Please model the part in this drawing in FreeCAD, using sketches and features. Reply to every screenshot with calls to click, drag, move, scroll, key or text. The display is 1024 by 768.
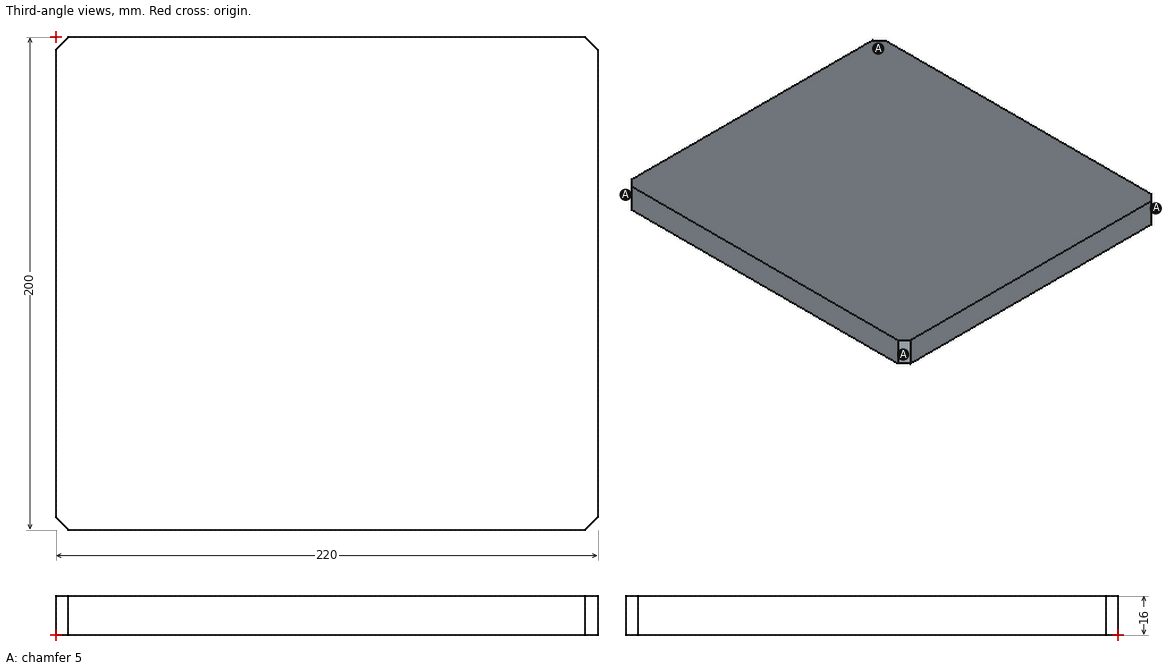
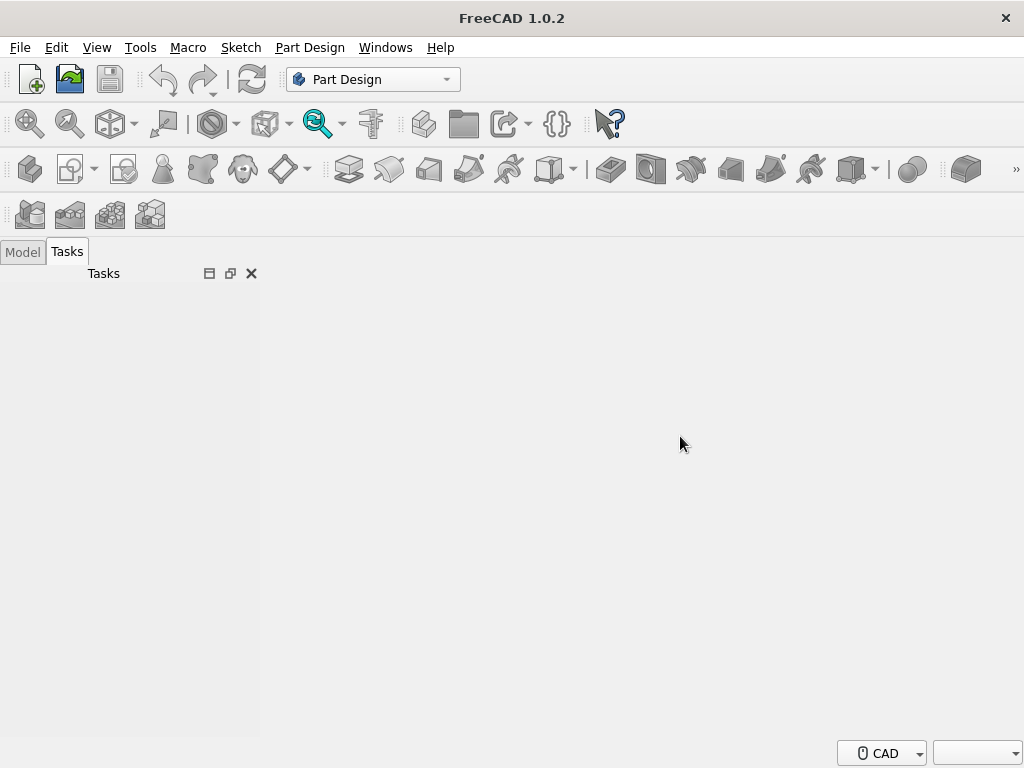
click(30, 80)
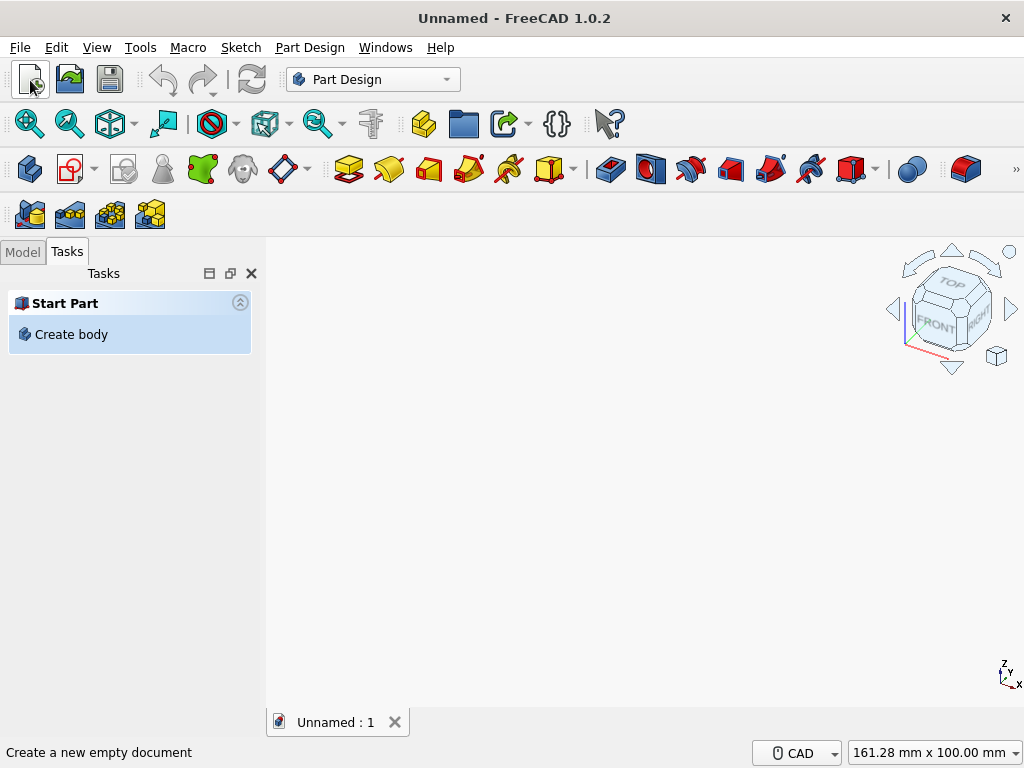
click(70, 170)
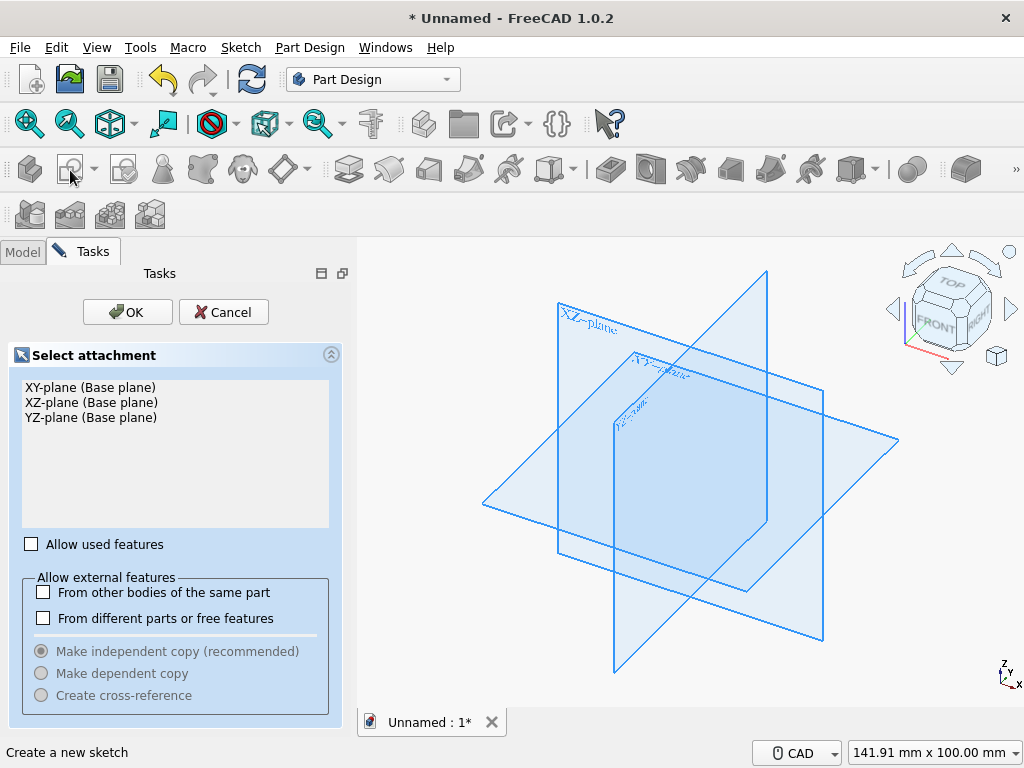
click(82, 388)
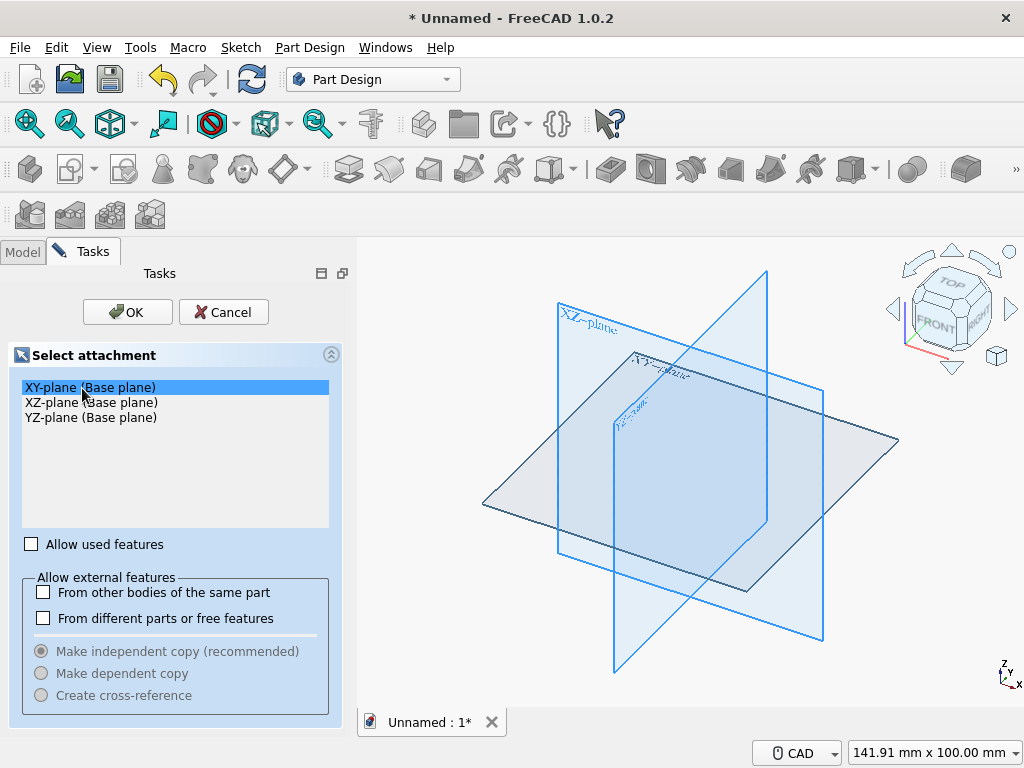
click(128, 312)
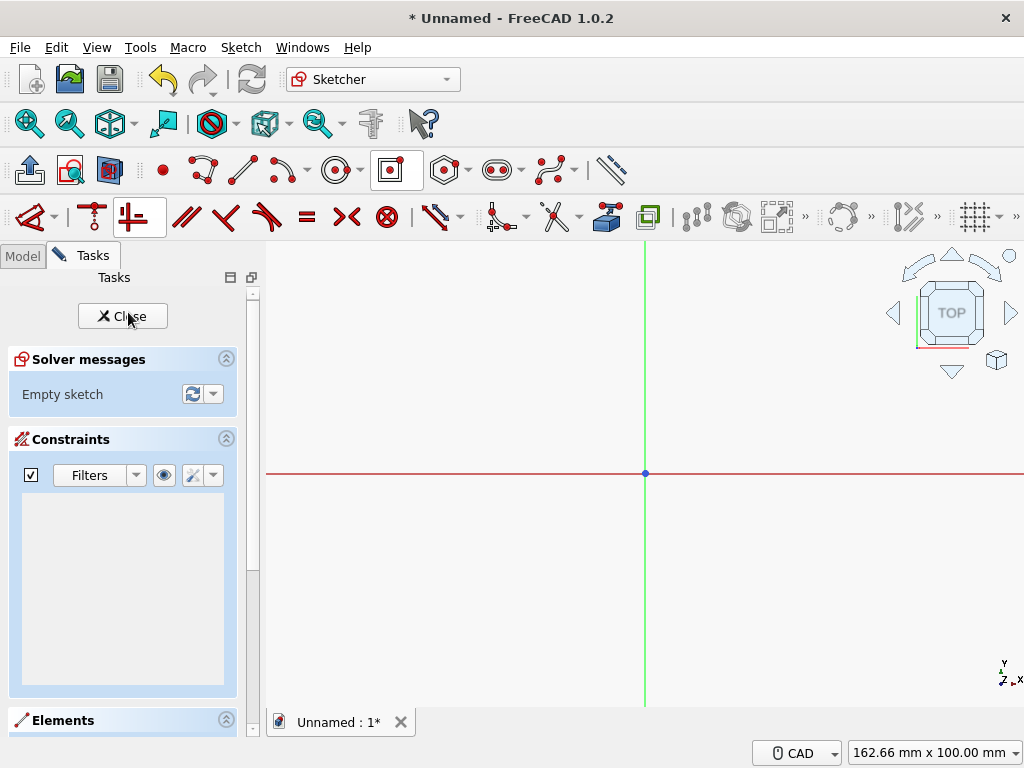
scroll(326, 273, down, 6)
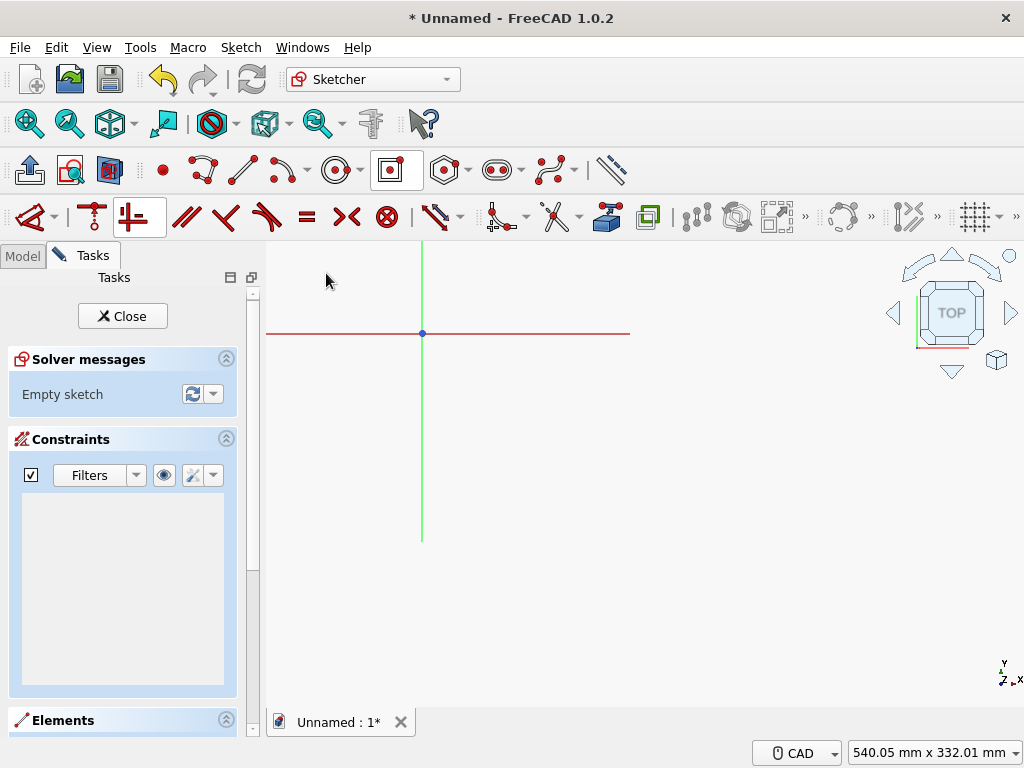
key(g)
key(r)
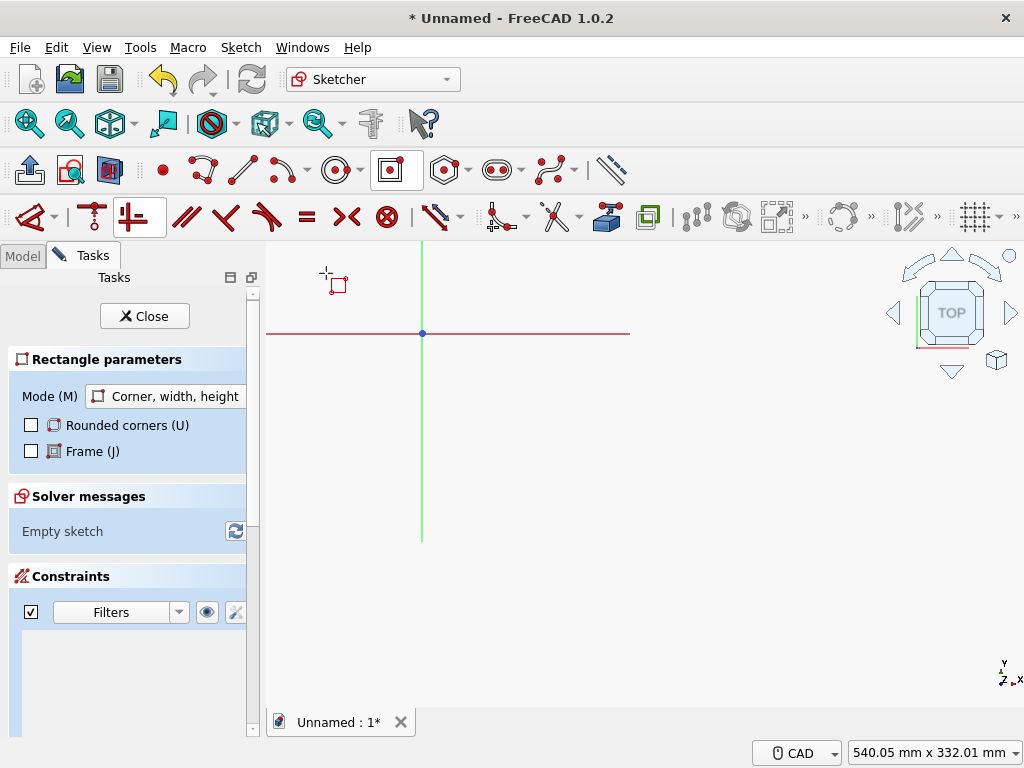
click(422, 334)
click(731, 614)
key(Escape)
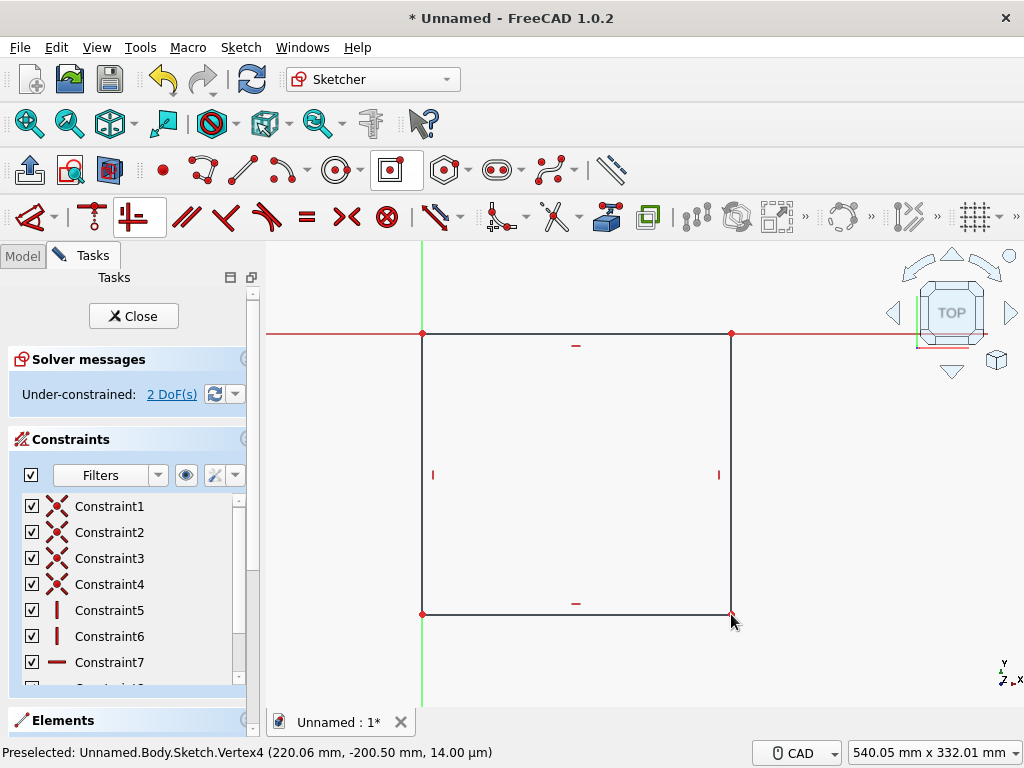
click(30, 218)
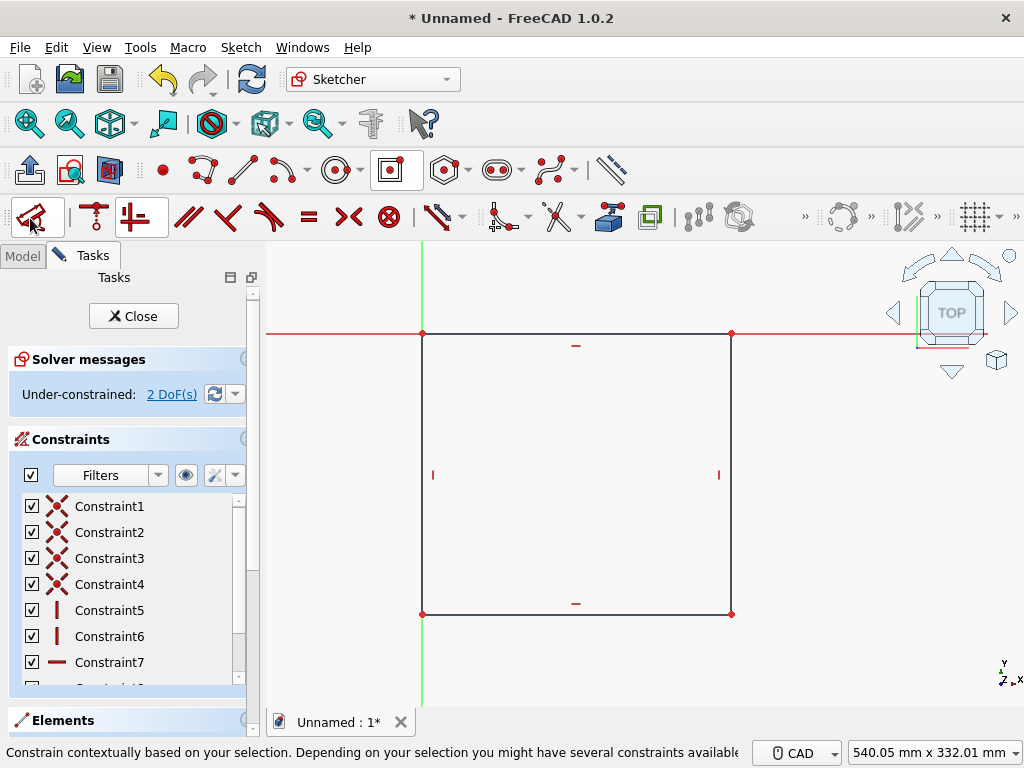
click(422, 418)
click(388, 474)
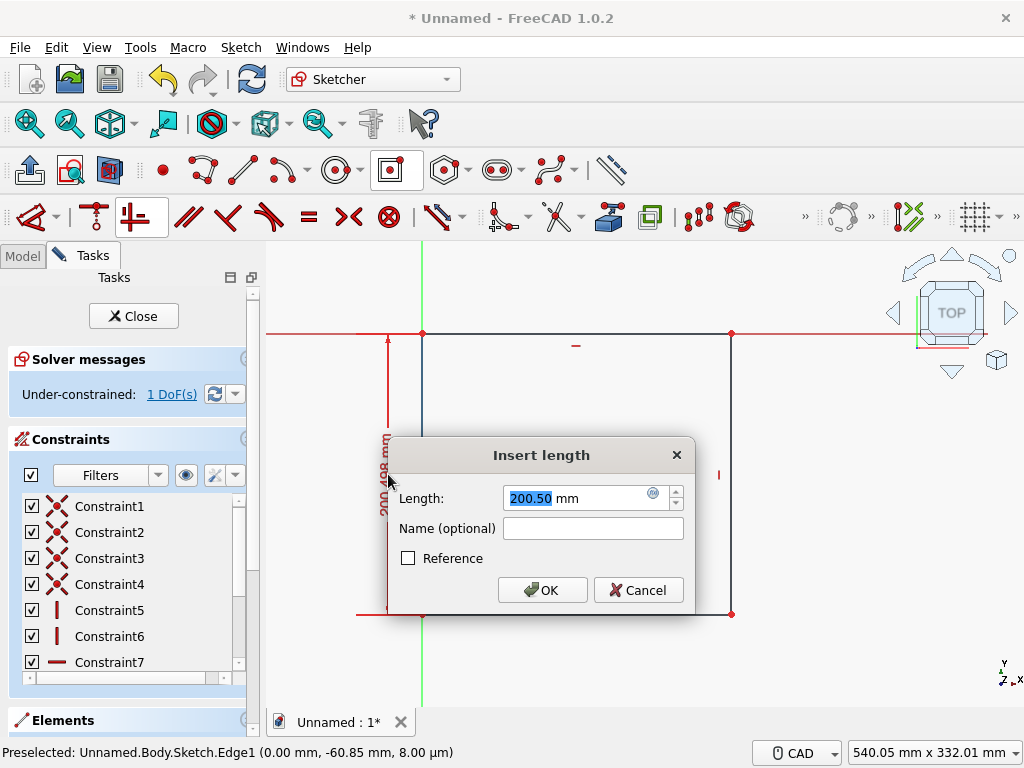
text(200)
key(Return)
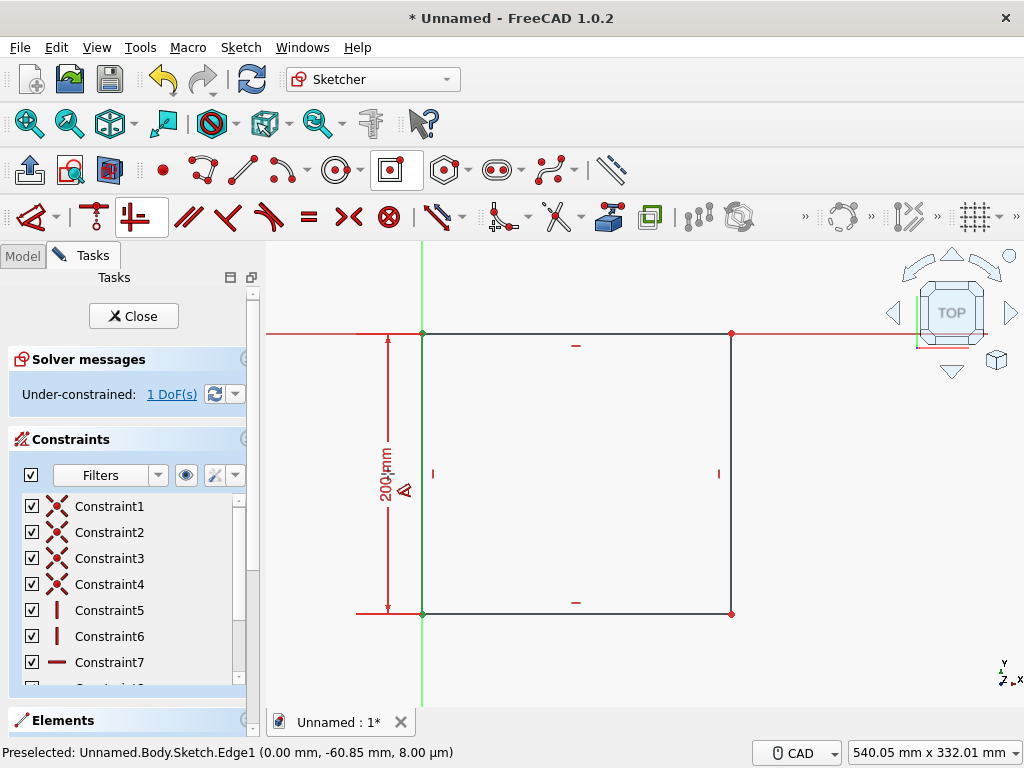
click(515, 614)
click(577, 648)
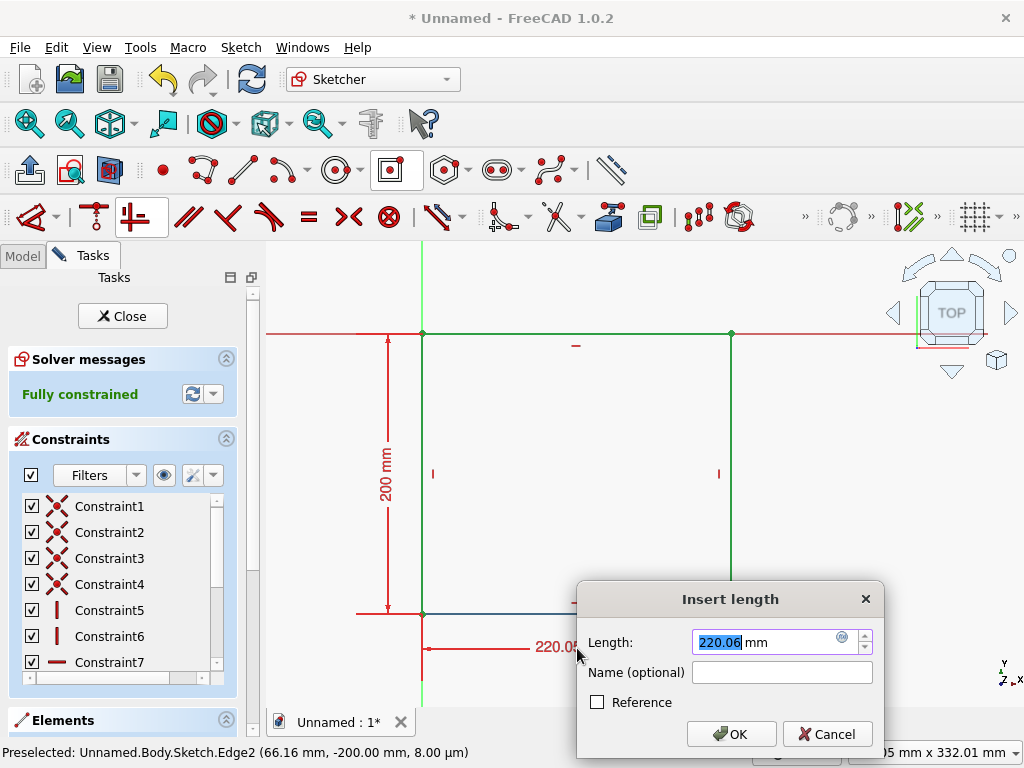
text(220)
key(Return)
key(Escape)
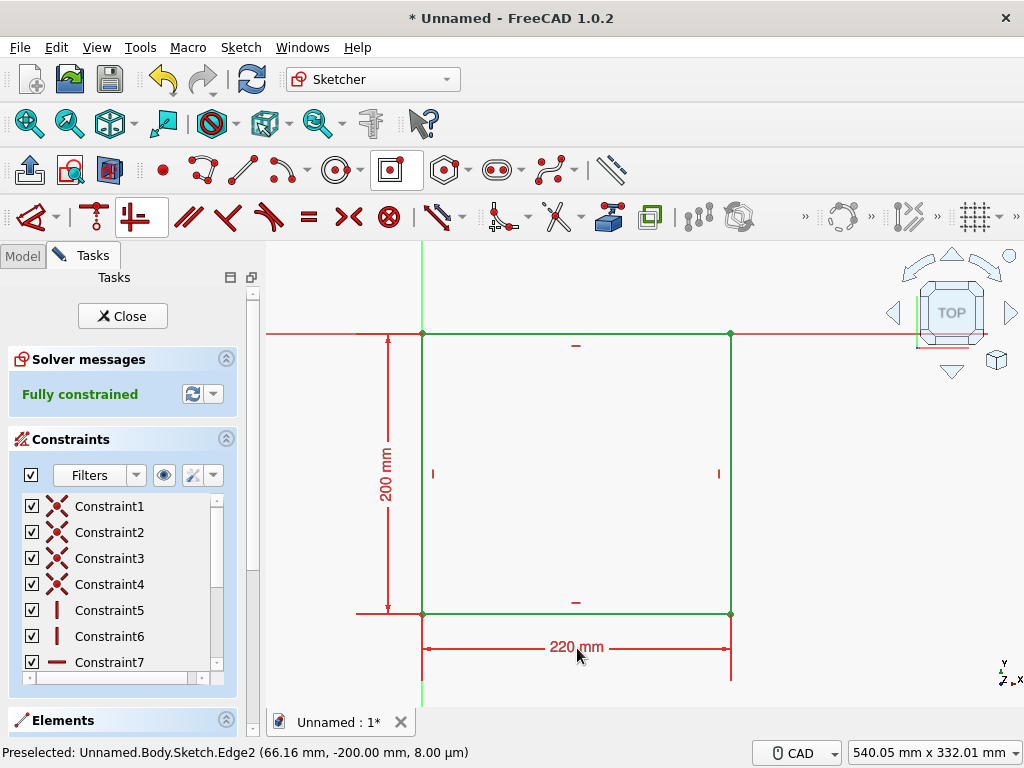
click(123, 316)